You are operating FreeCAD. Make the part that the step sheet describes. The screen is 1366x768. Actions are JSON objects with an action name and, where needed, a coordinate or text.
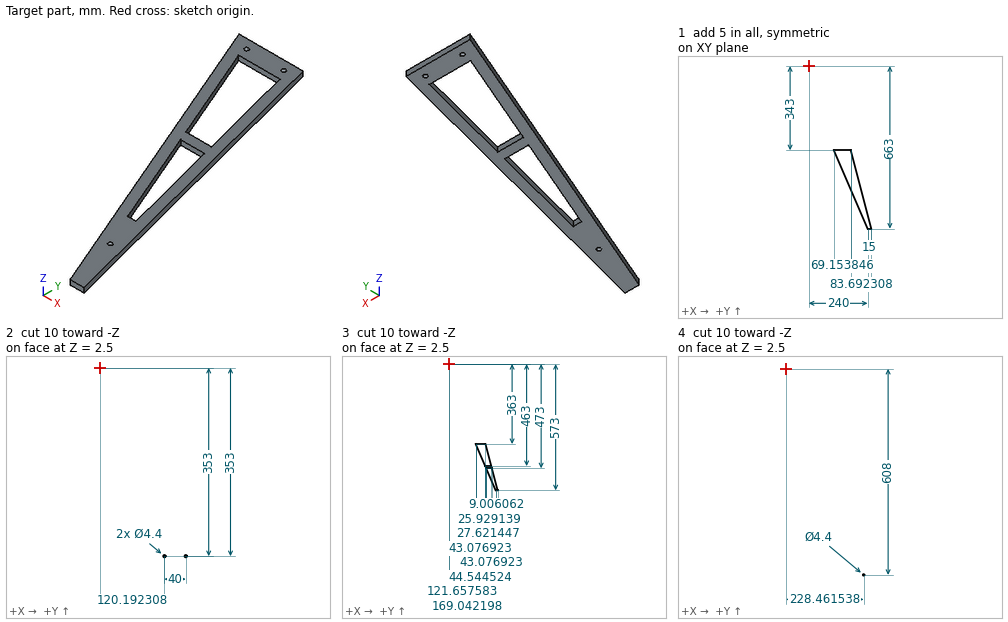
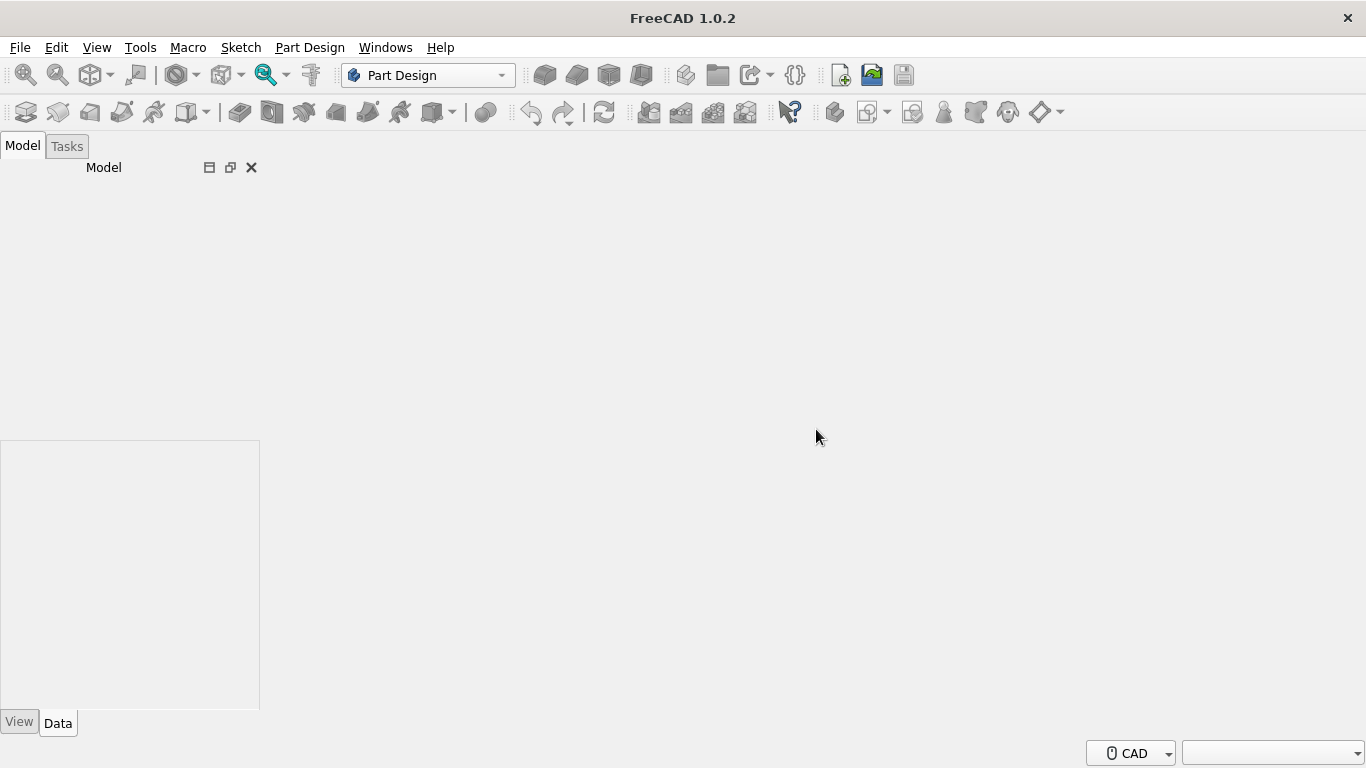
{"action": "left_click", "coordinate": [840, 76]}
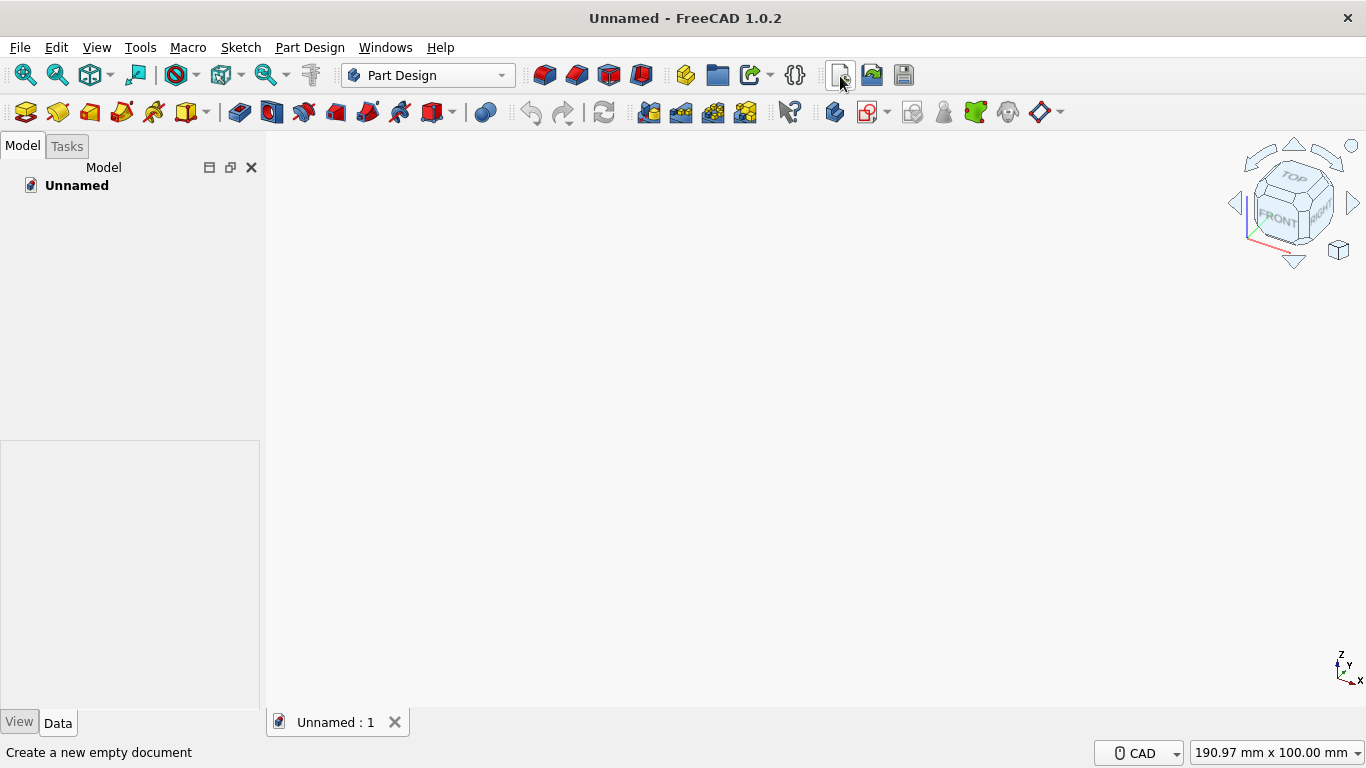
{"action": "left_click", "coordinate": [868, 112]}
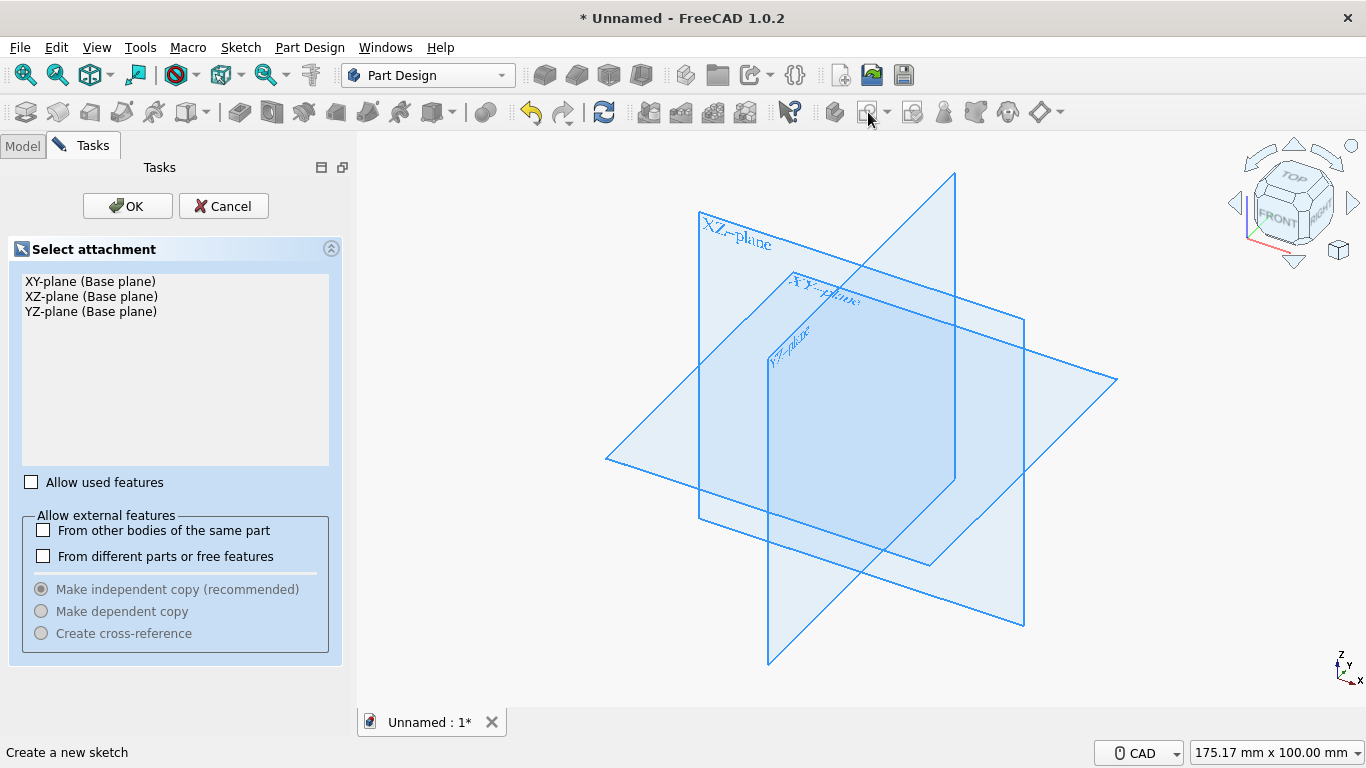
{"action": "left_click", "coordinate": [82, 282]}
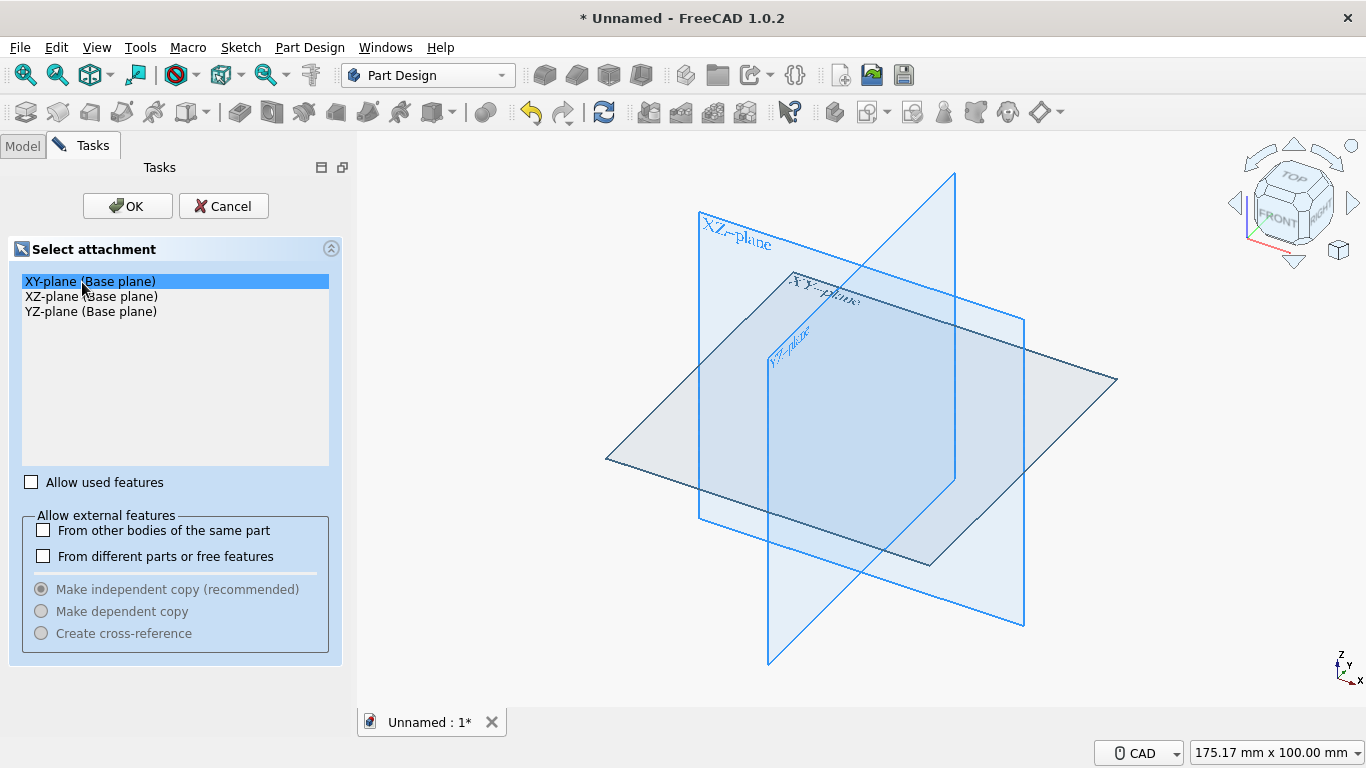
{"action": "left_click", "coordinate": [128, 206]}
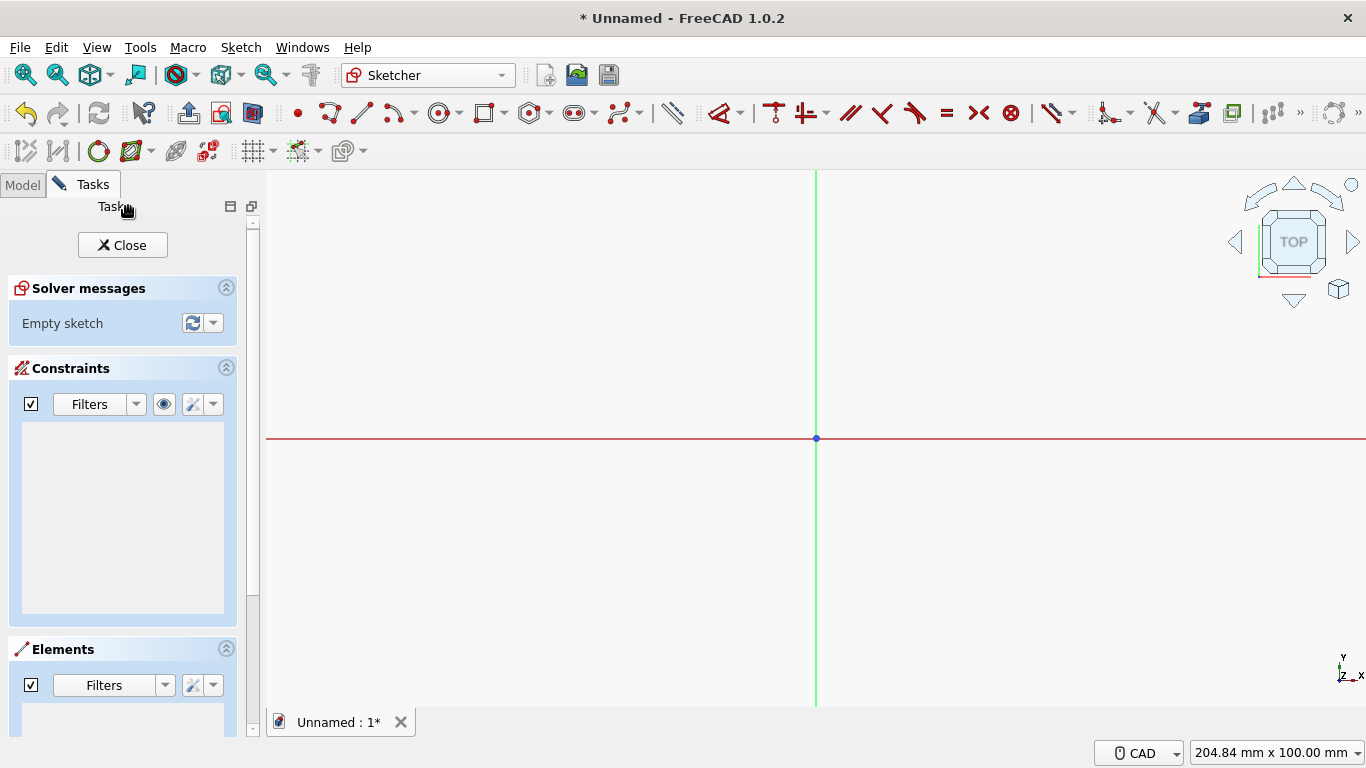
{"action": "scroll", "coordinate": [672, 261], "scroll_direction": "down", "scroll_amount": 12}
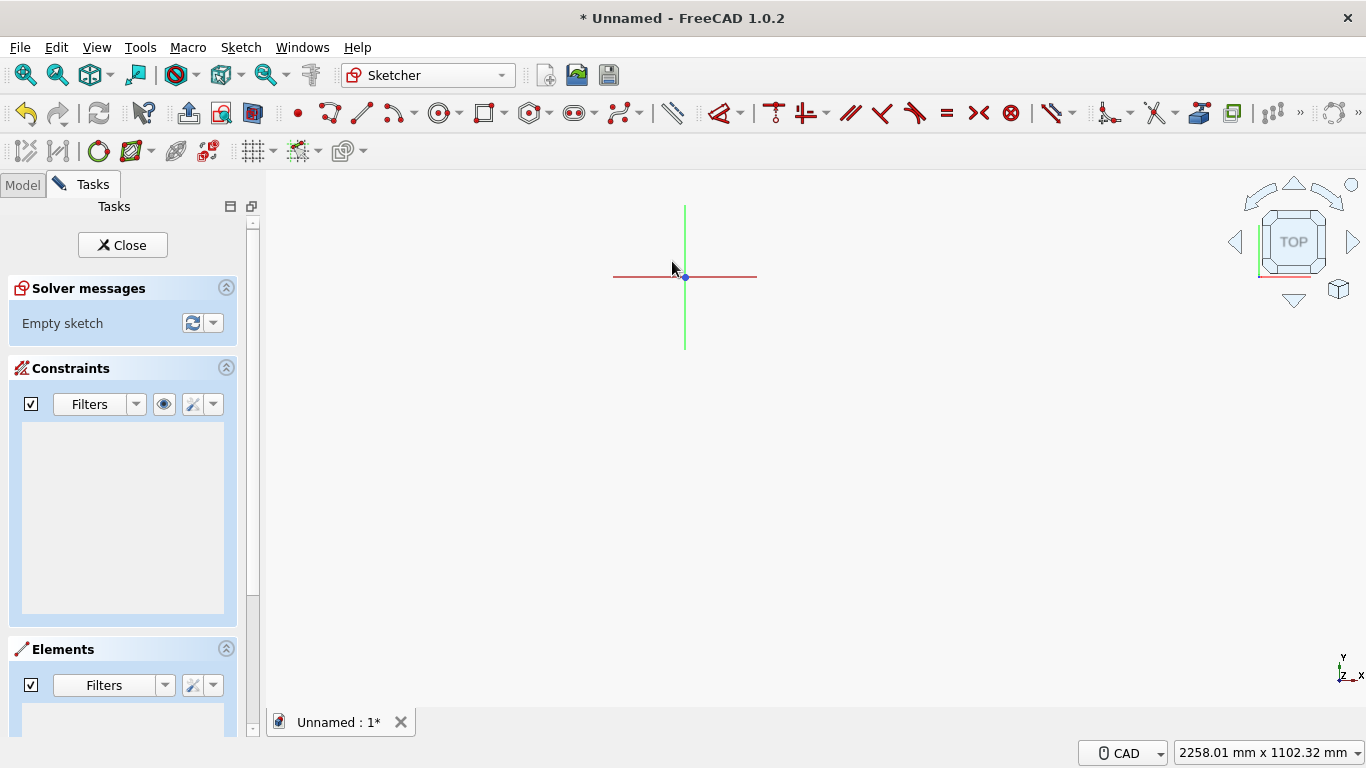
{"action": "key", "text": "g m"}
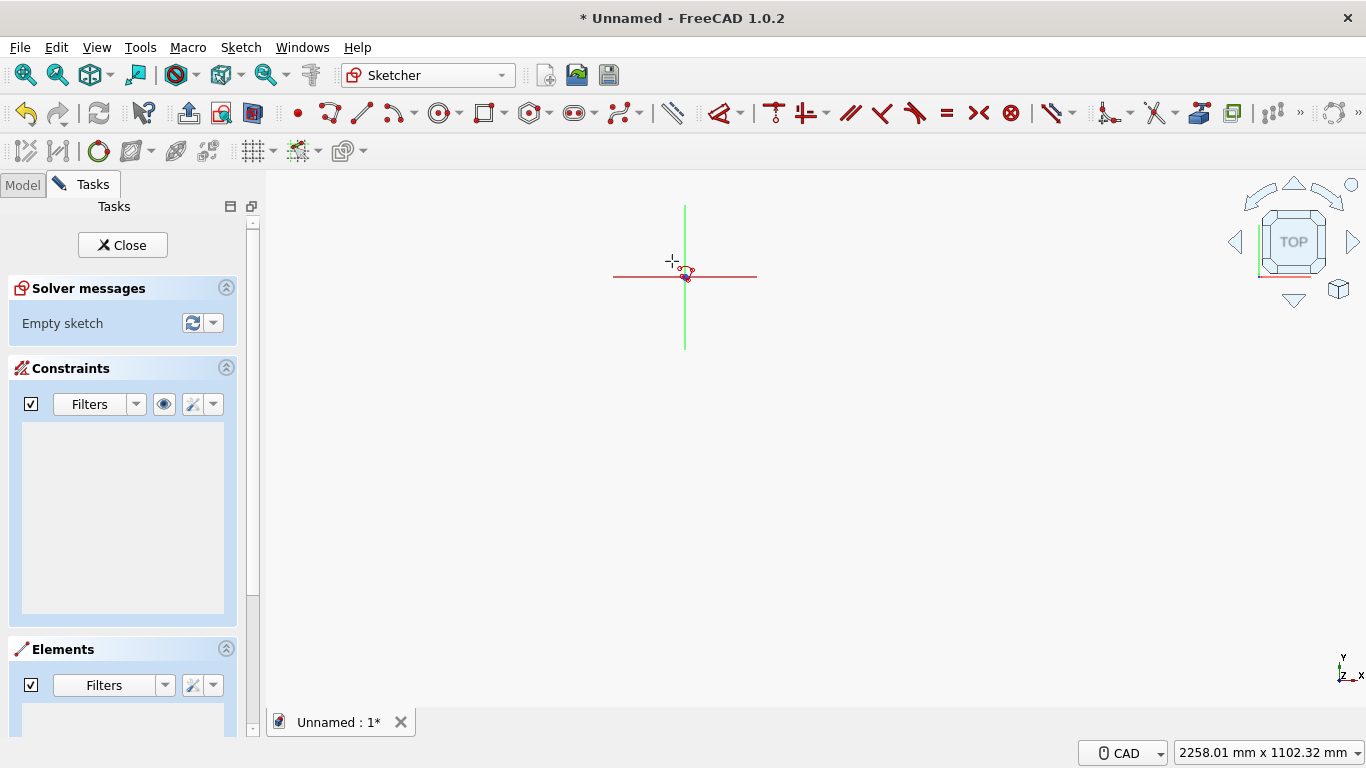
{"action": "left_click", "coordinate": [735, 444]}
{"action": "left_click", "coordinate": [802, 600]}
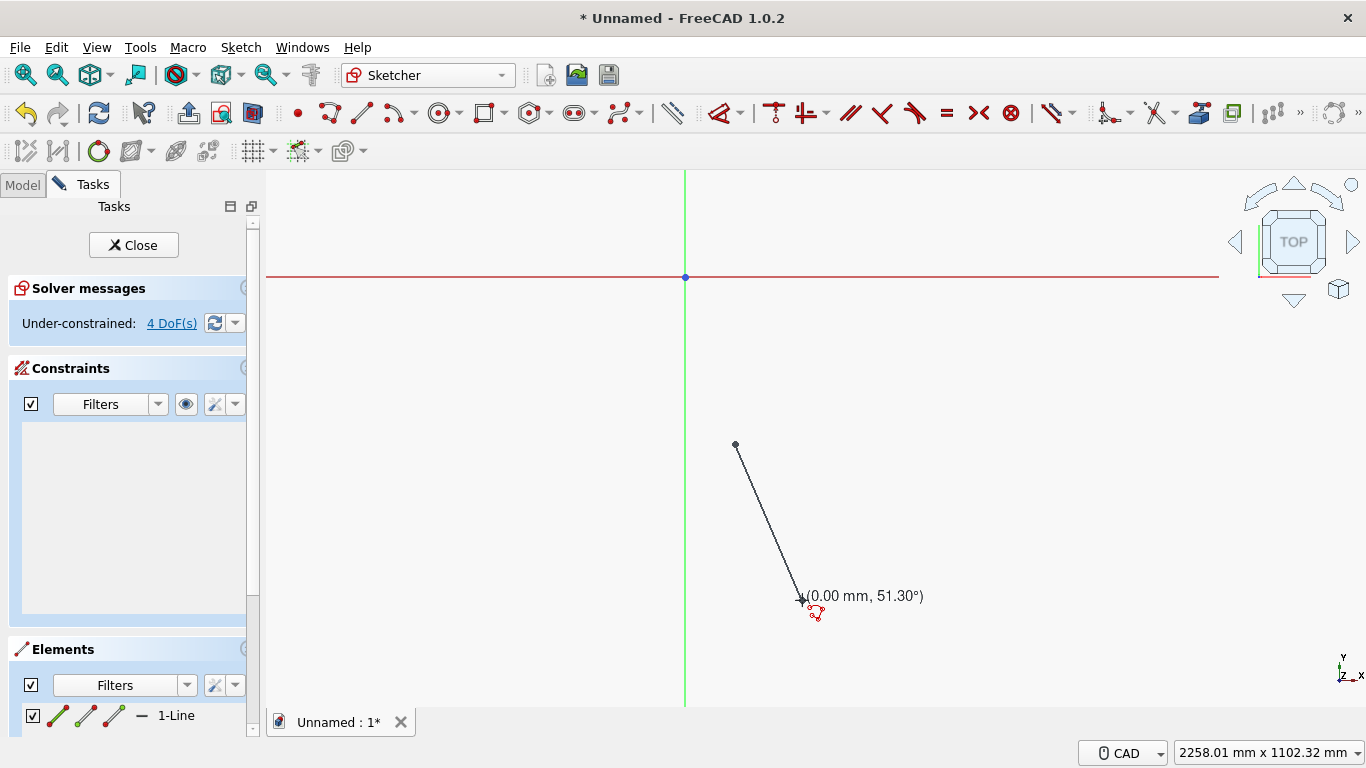
{"action": "scroll", "coordinate": [810, 600], "scroll_direction": "up", "scroll_amount": 4}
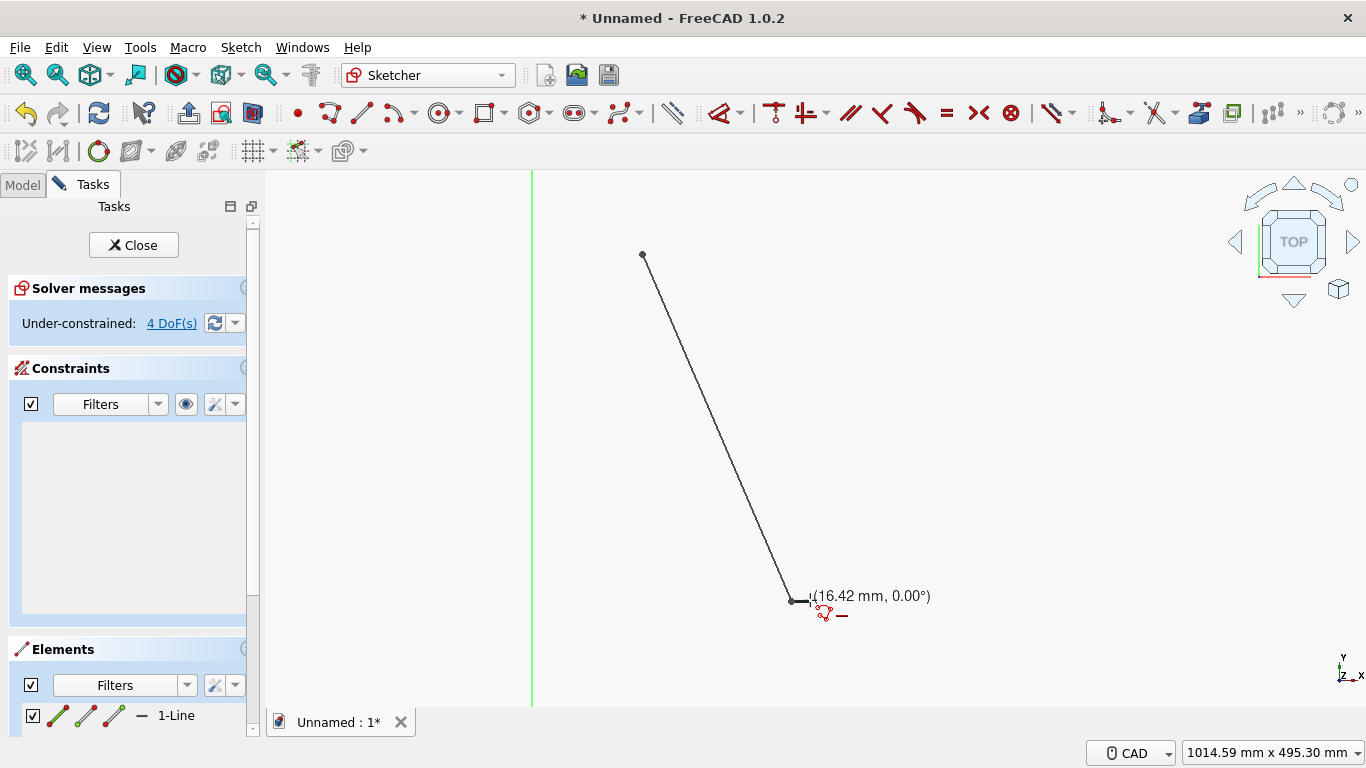
{"action": "left_click", "coordinate": [809, 599]}
{"action": "left_click", "coordinate": [718, 253]}
{"action": "left_click", "coordinate": [642, 254]}
{"action": "key", "text": "Escape"}
{"action": "key", "text": "Escape"}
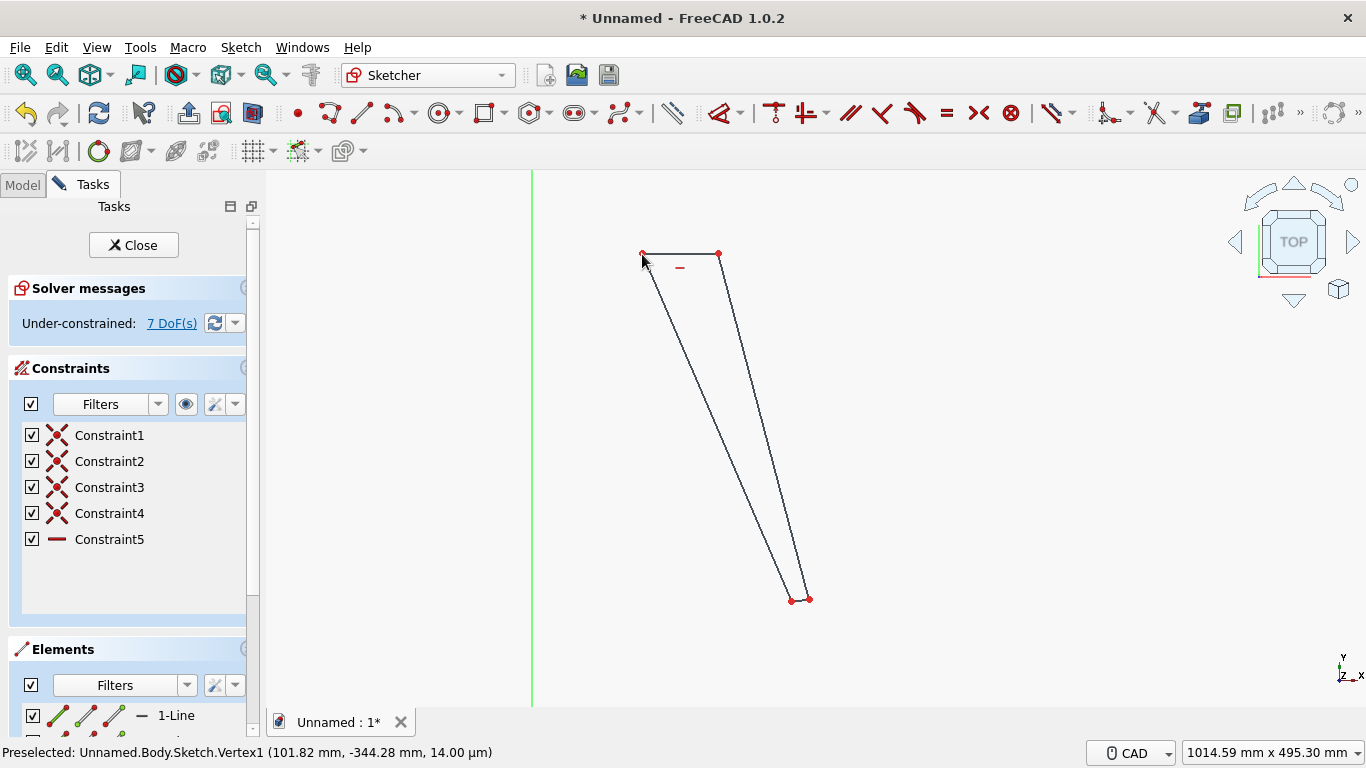
{"action": "scroll", "coordinate": [800, 601], "scroll_direction": "up", "scroll_amount": 3}